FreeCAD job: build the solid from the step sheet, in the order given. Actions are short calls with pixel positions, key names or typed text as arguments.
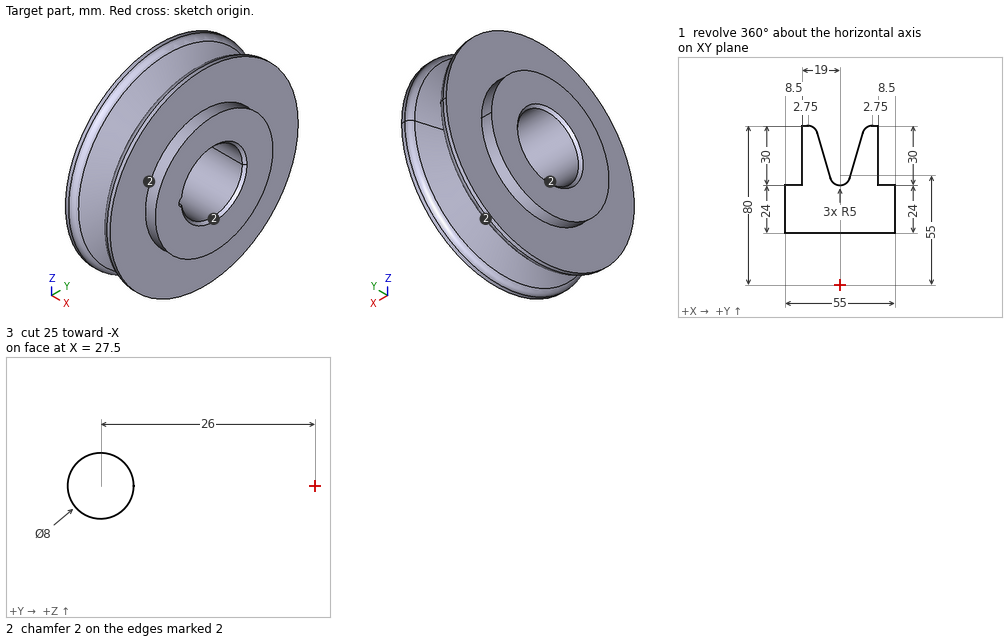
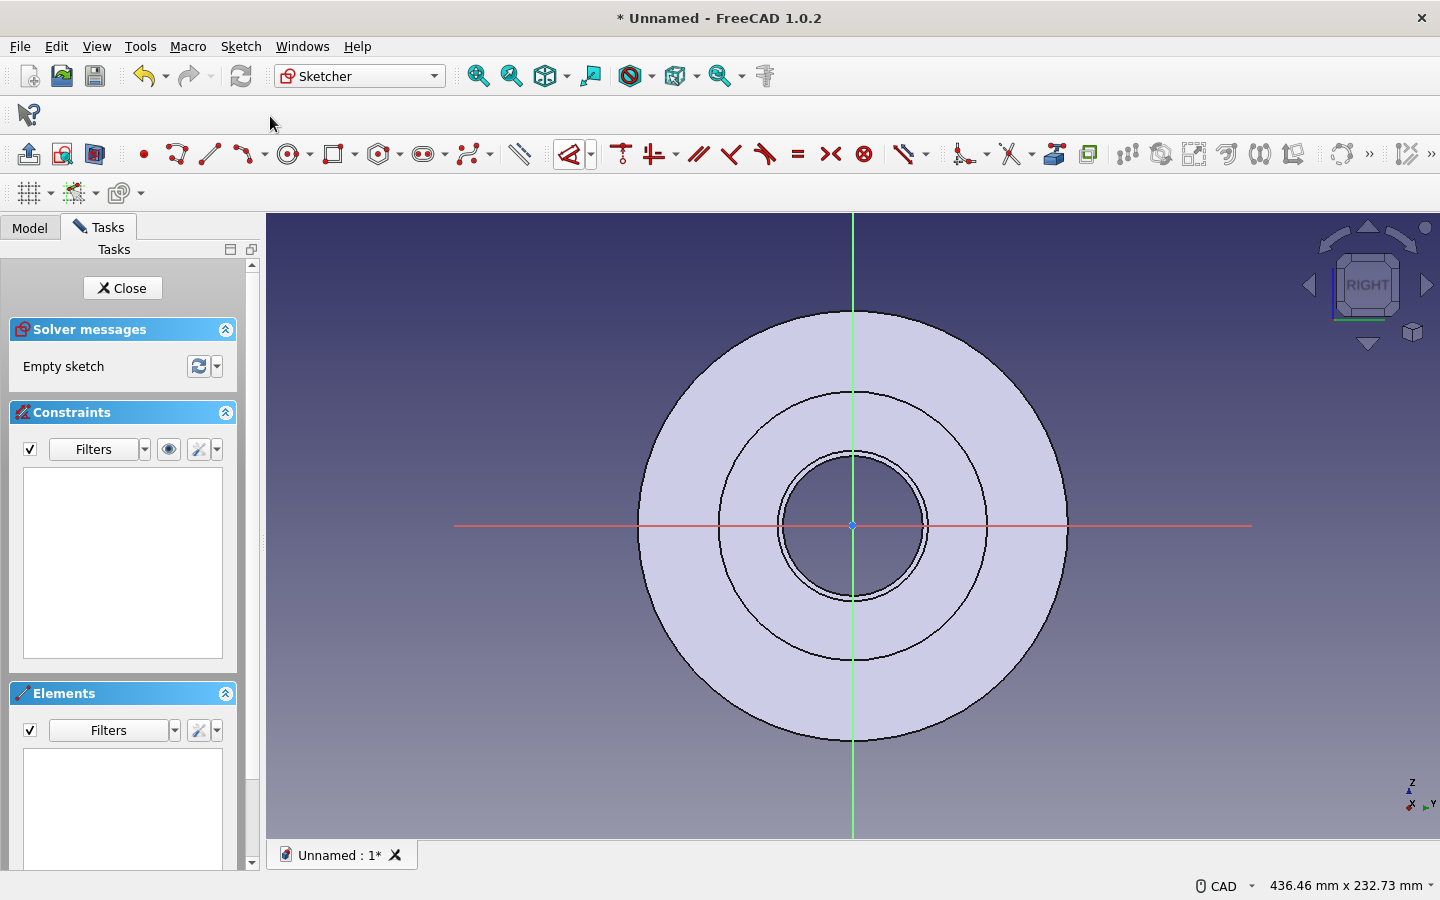
scroll(783, 526, up, 15)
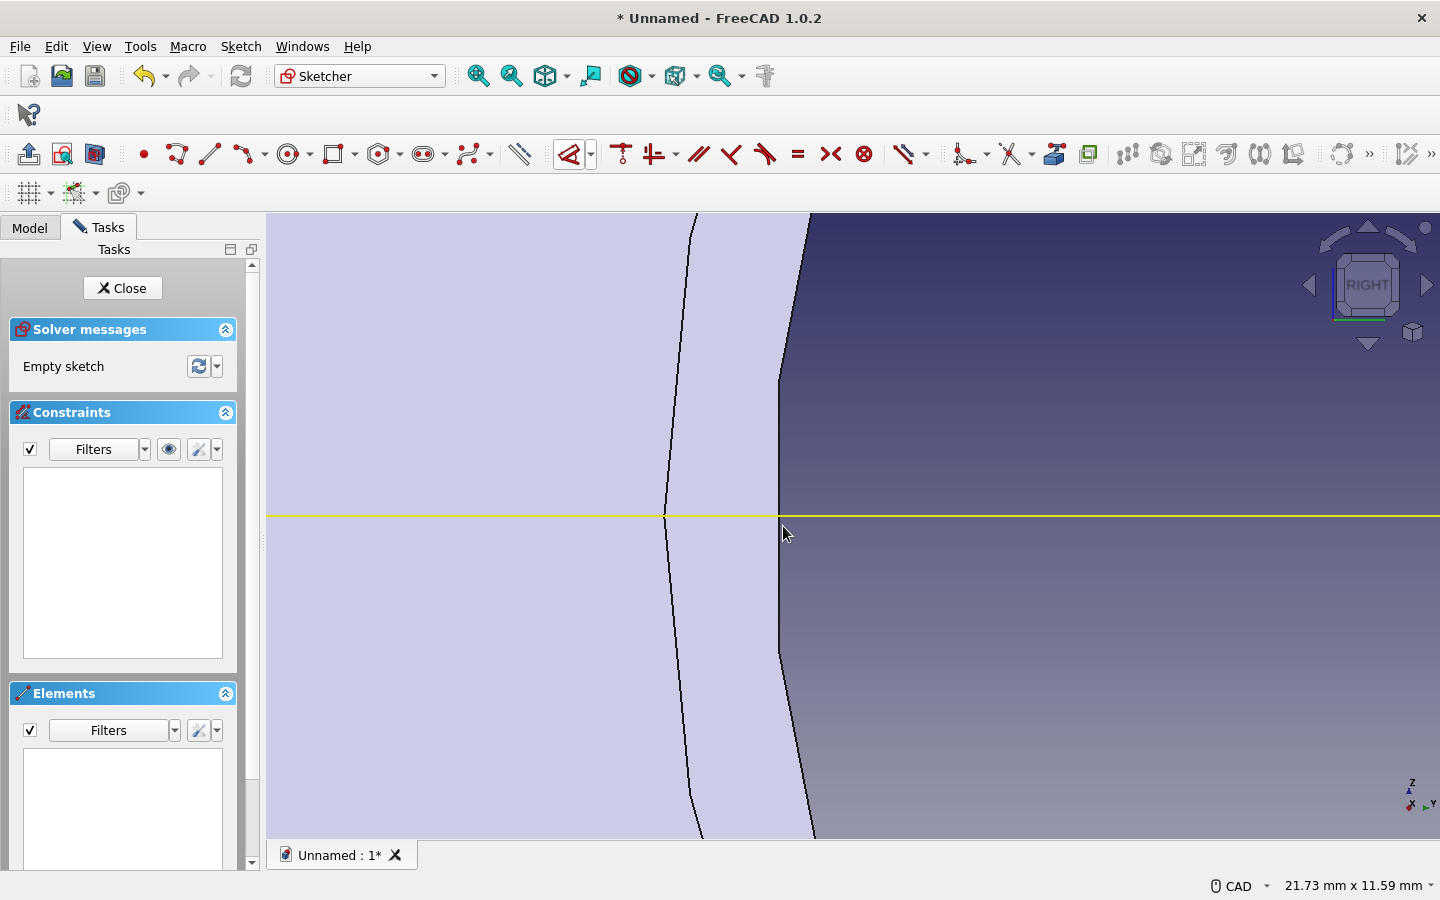
key(g)
key(c)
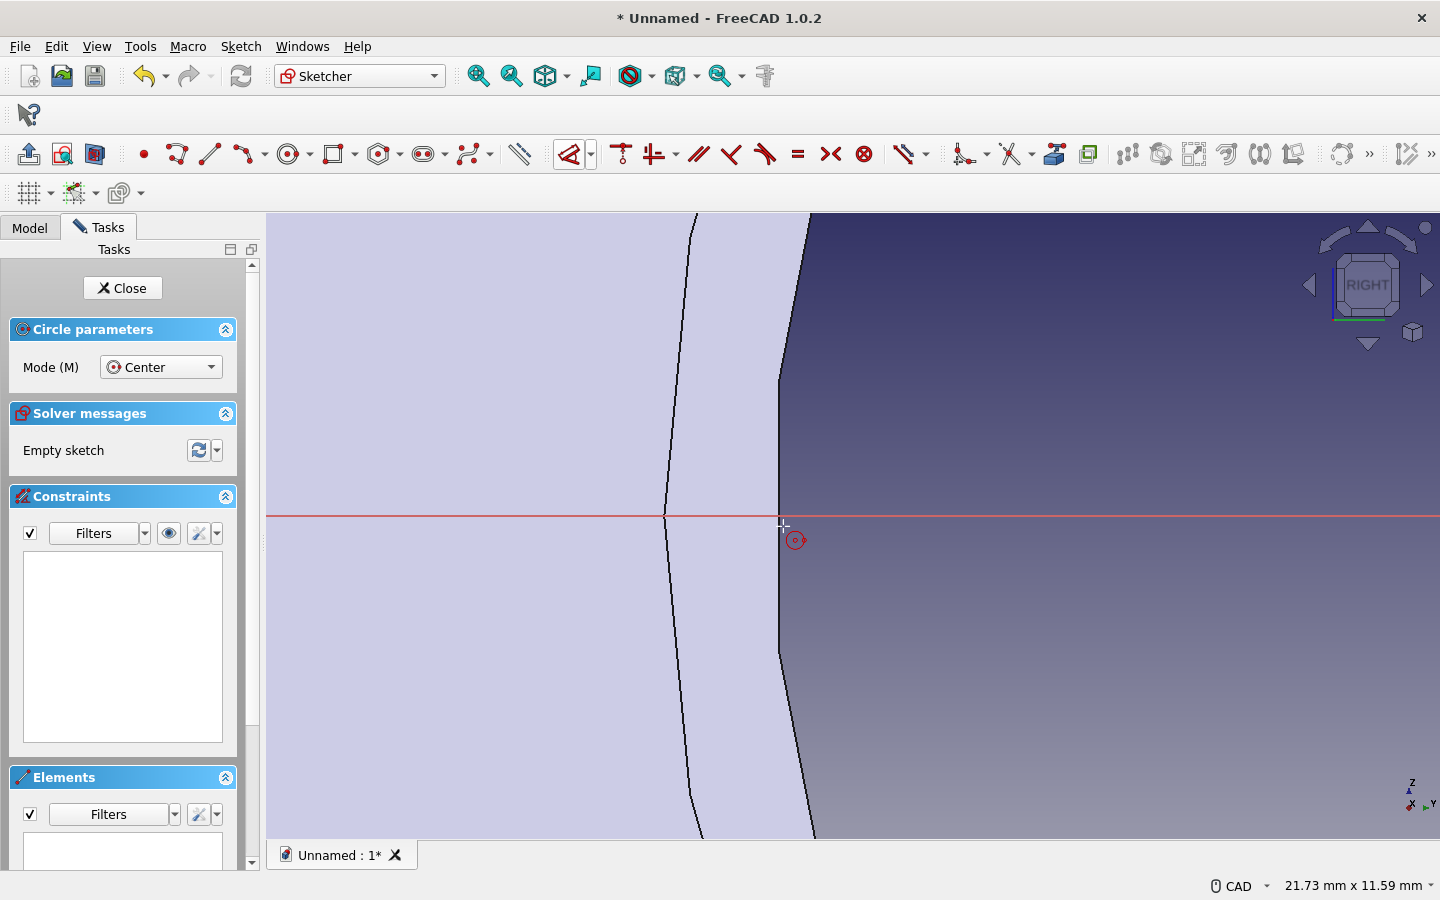
click(772, 516)
click(925, 364)
key(Escape)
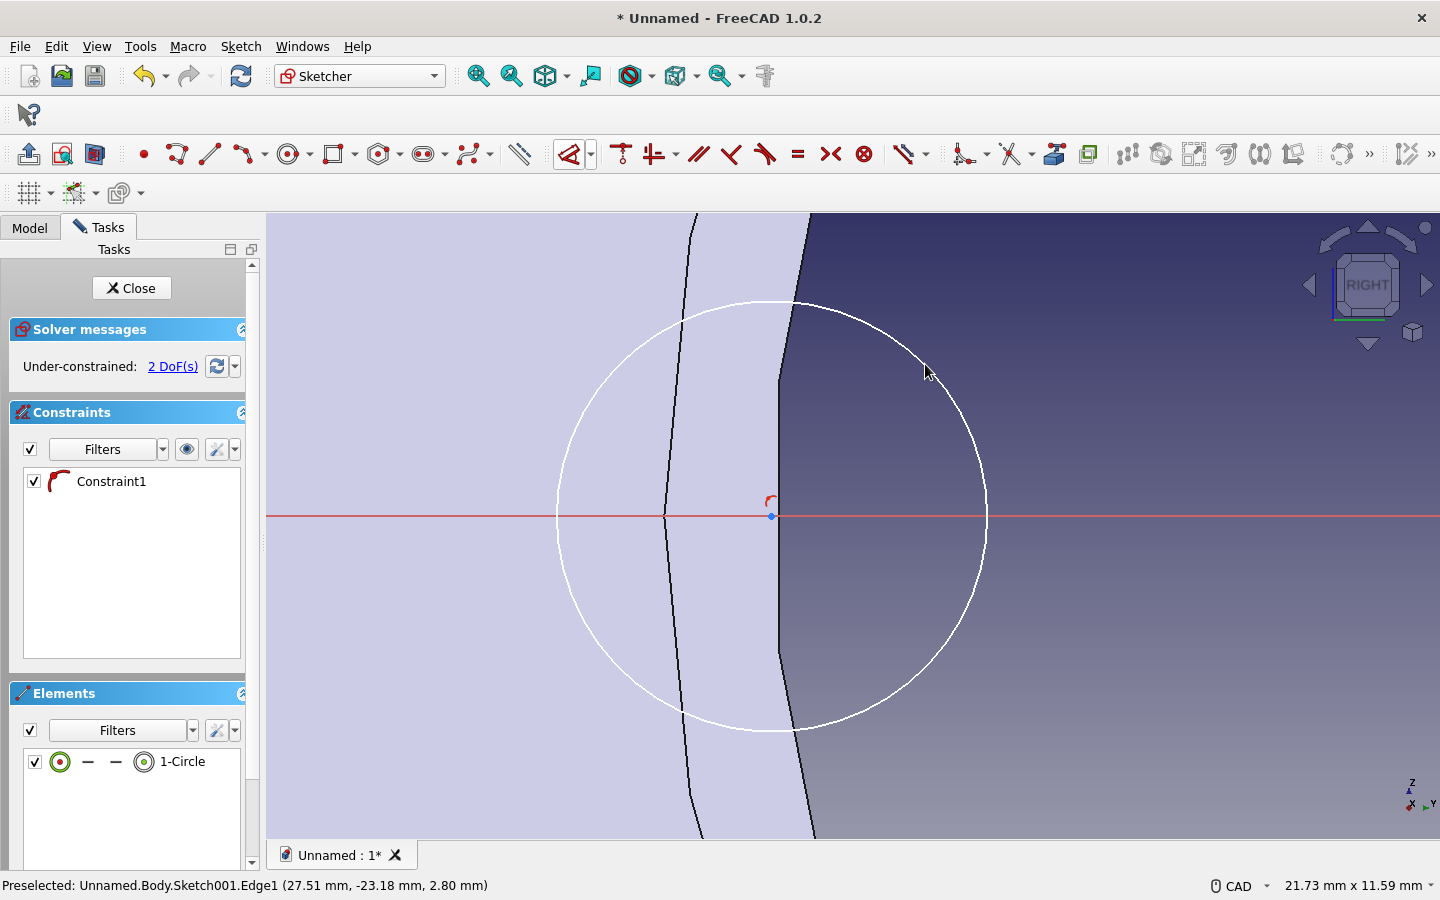
click(924, 364)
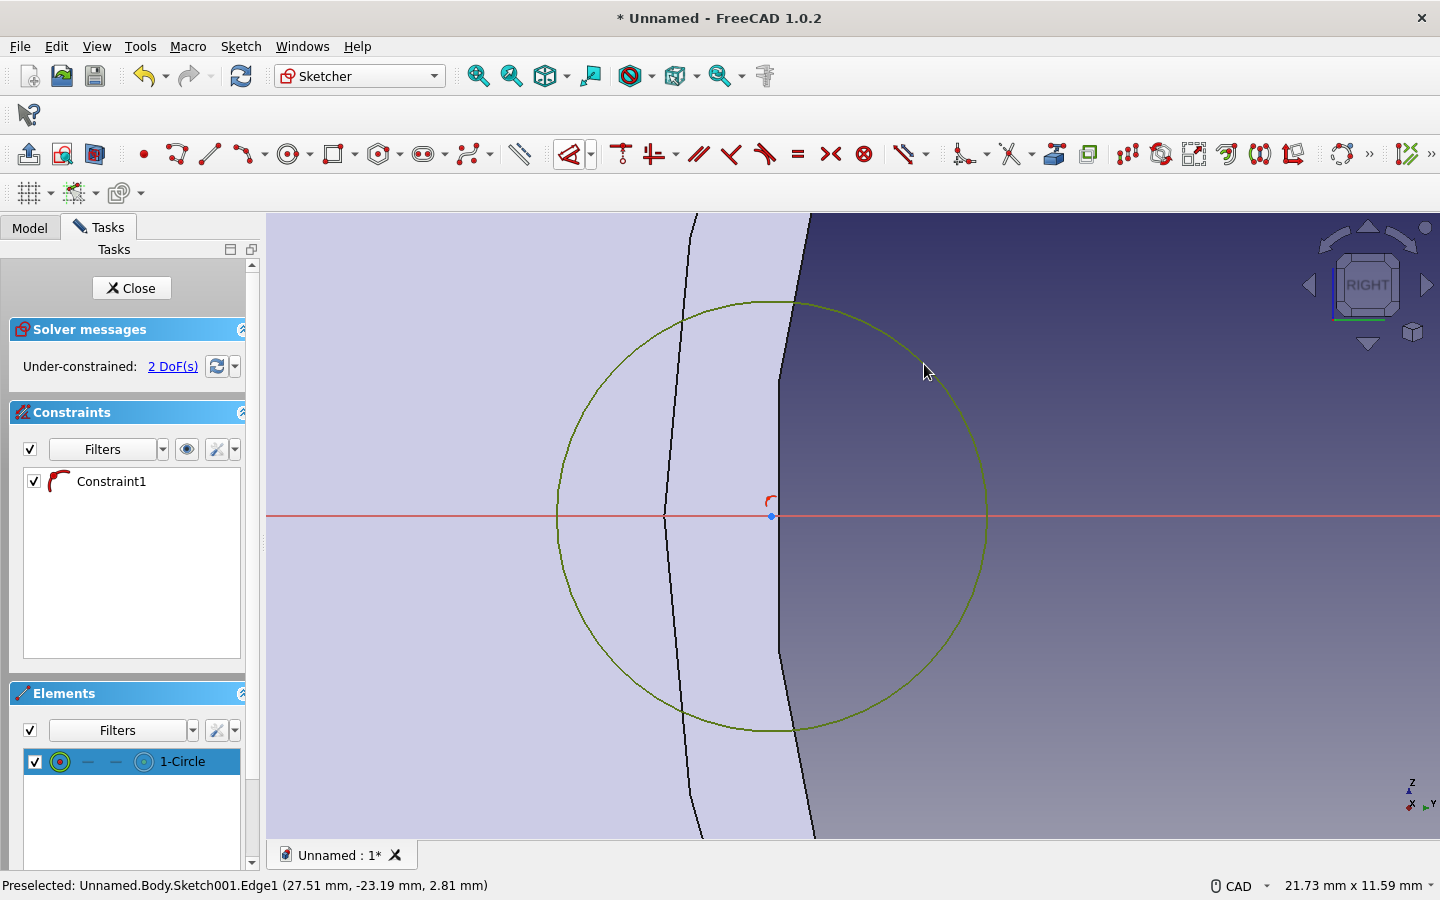
key(k)
key(o)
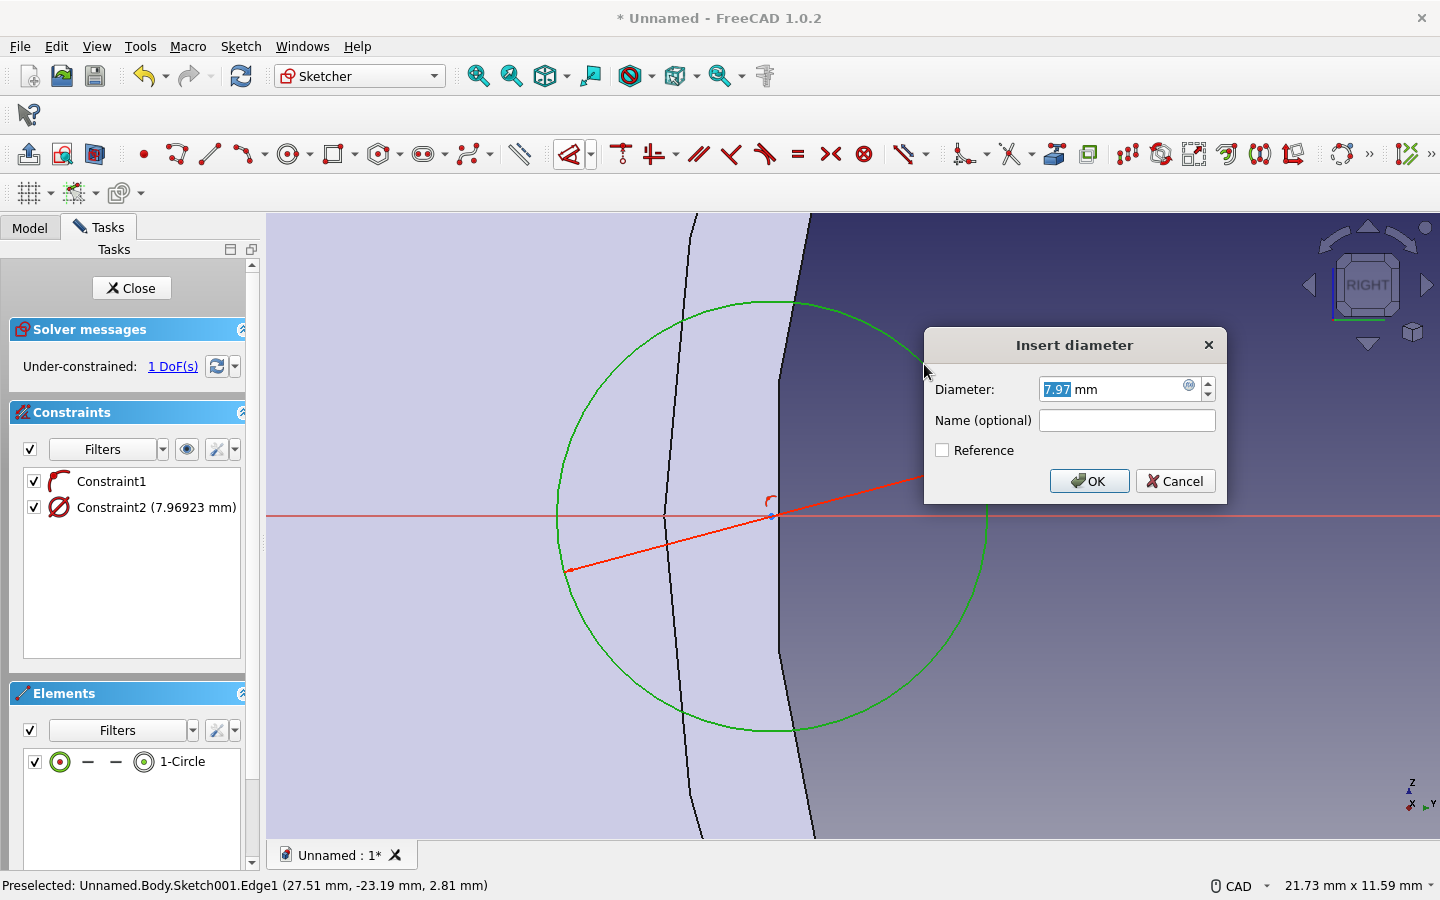
text(8)
key(Return)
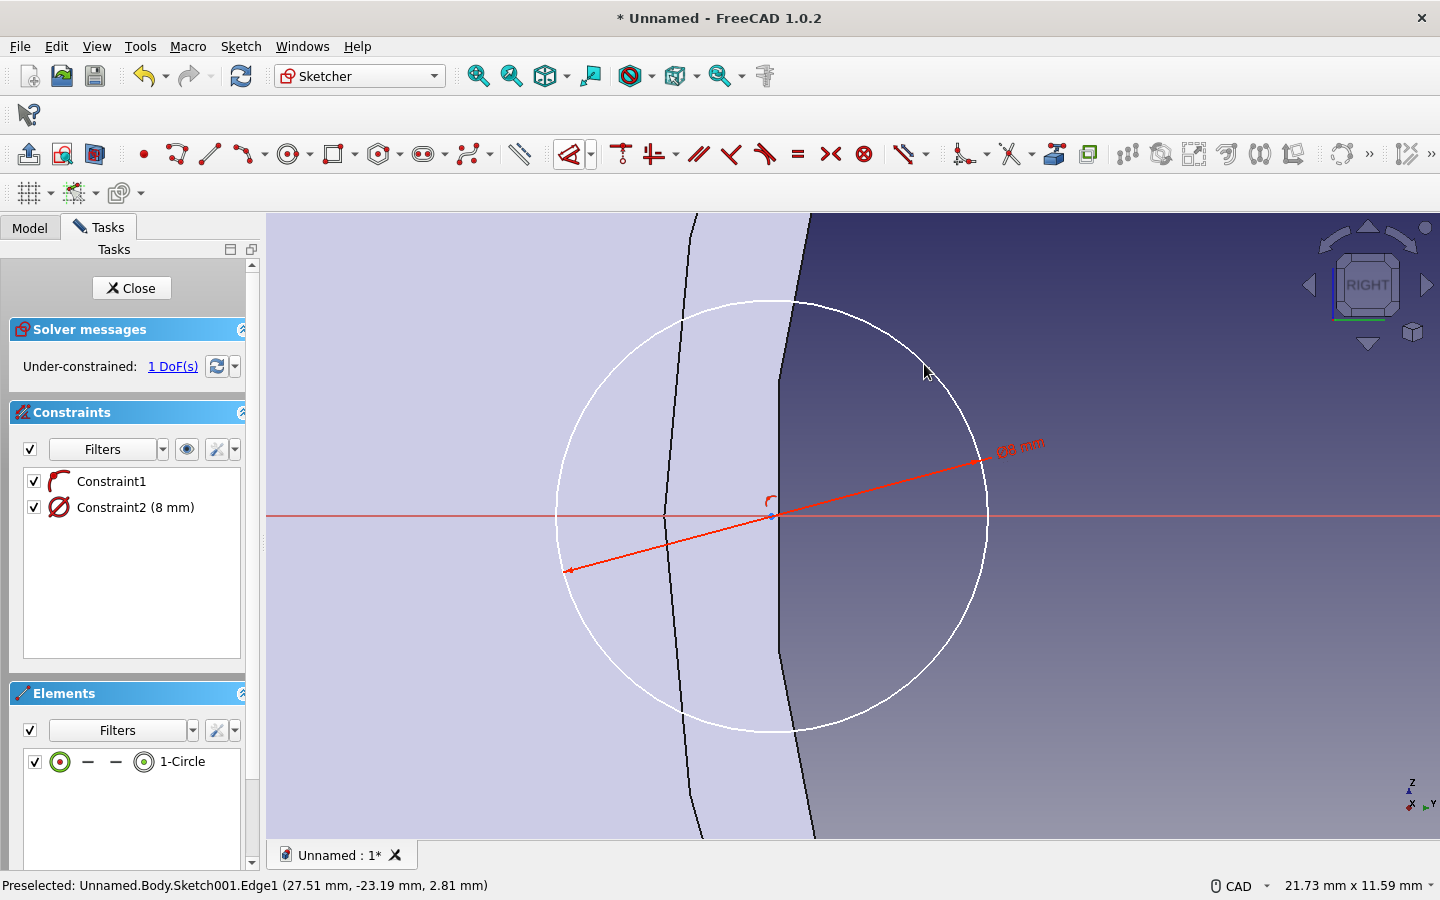
click(772, 516)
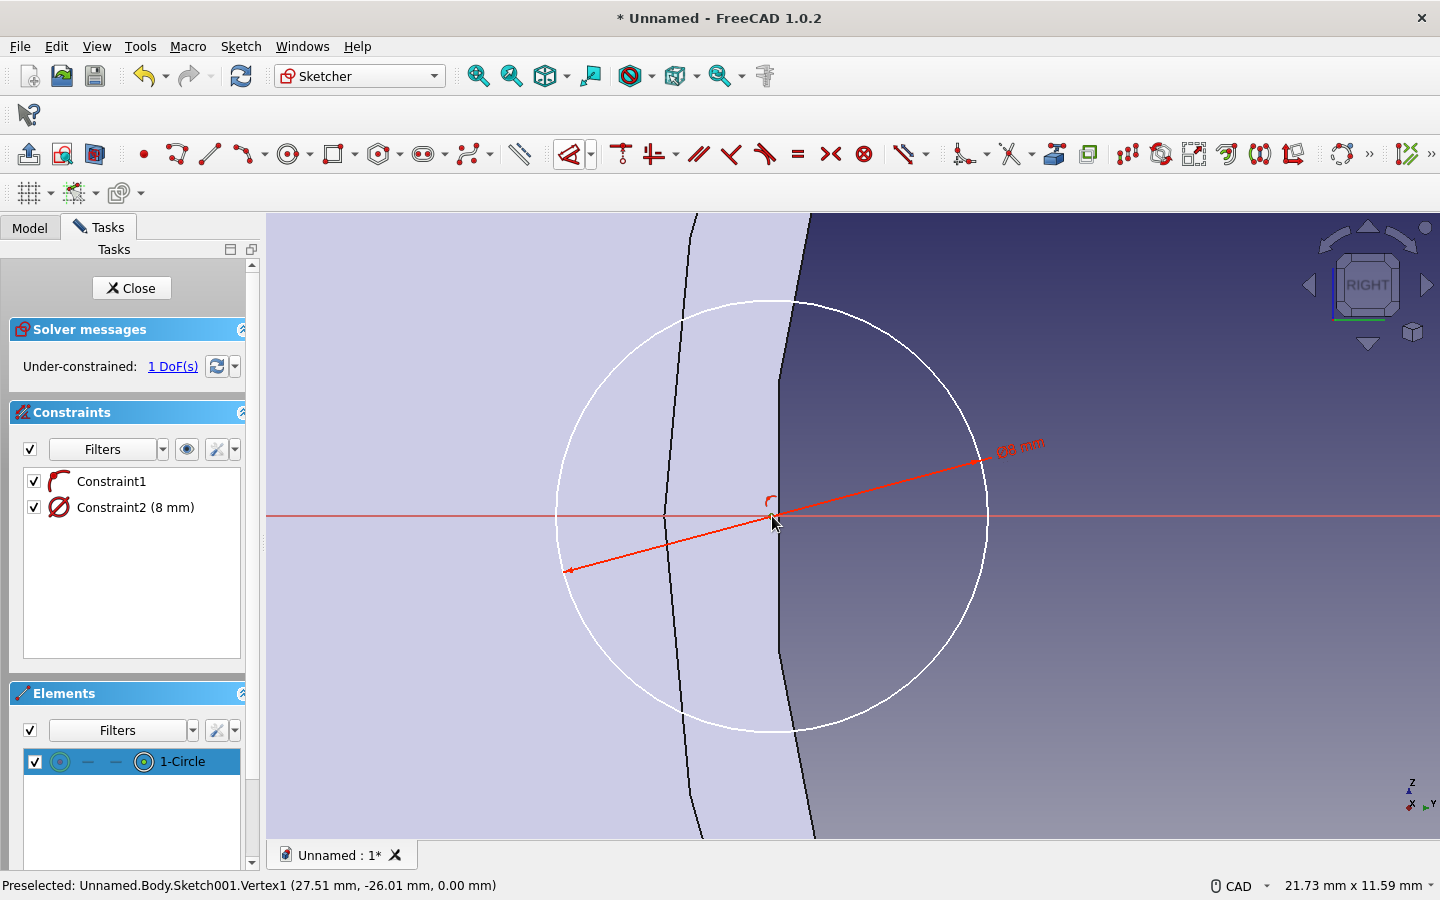
click(590, 154)